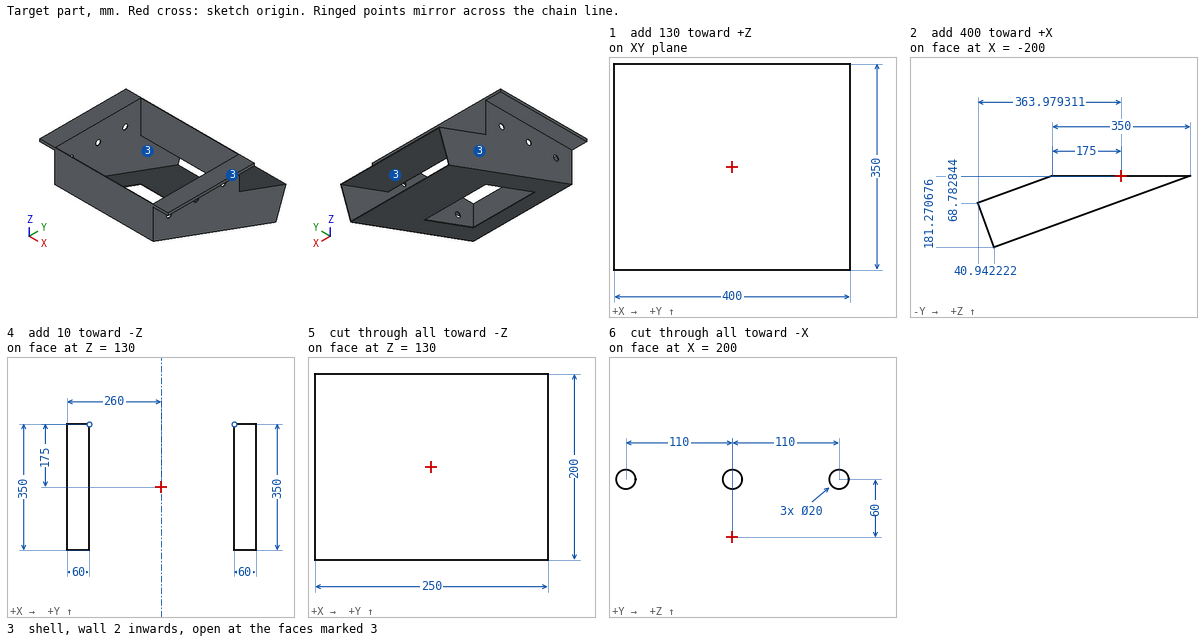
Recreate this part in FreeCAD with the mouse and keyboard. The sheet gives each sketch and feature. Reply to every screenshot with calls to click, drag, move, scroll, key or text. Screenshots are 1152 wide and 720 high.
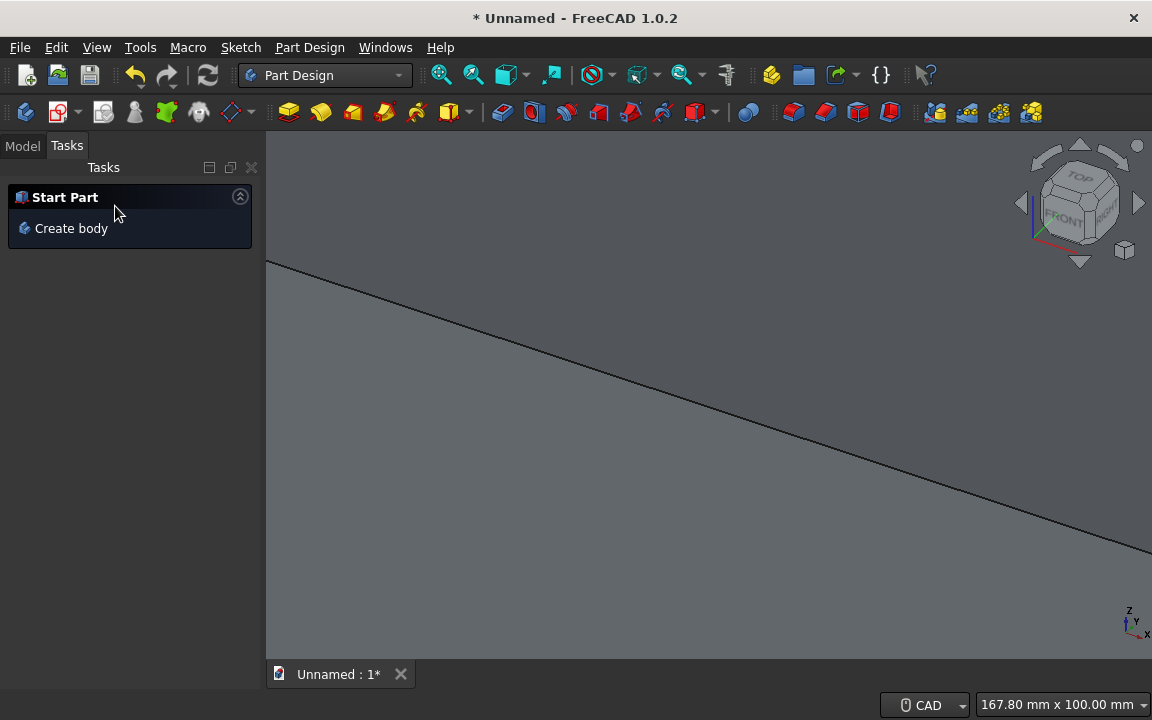
key(v)
key(f)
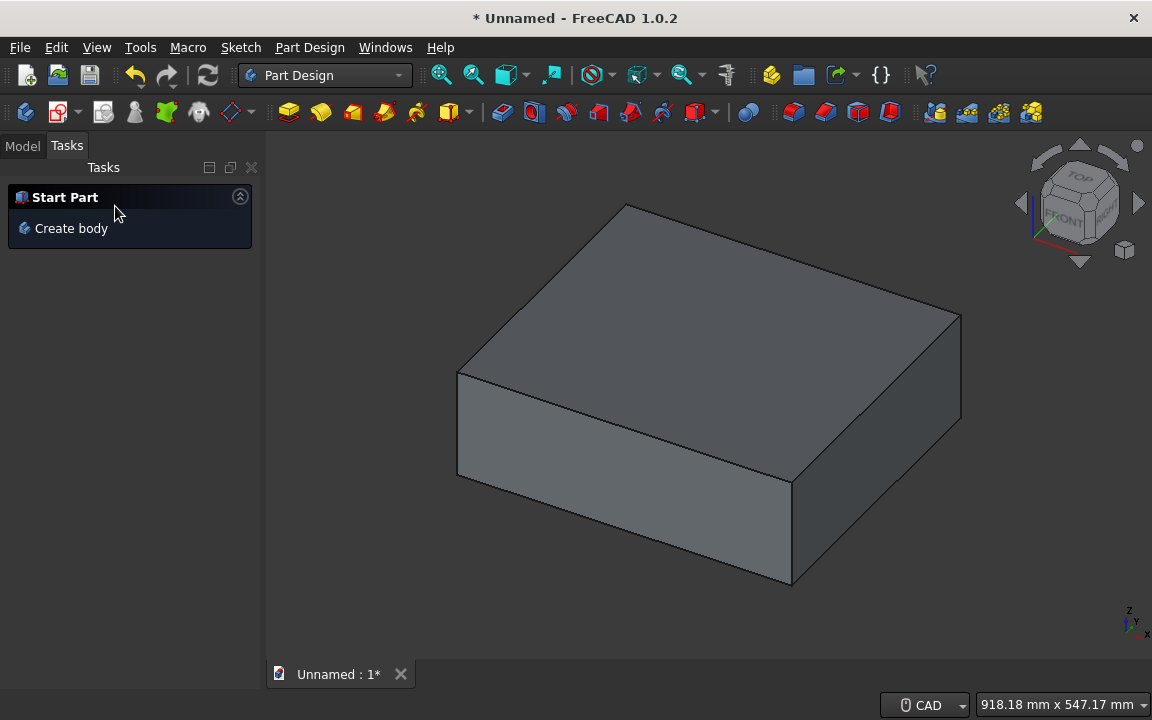
key(6)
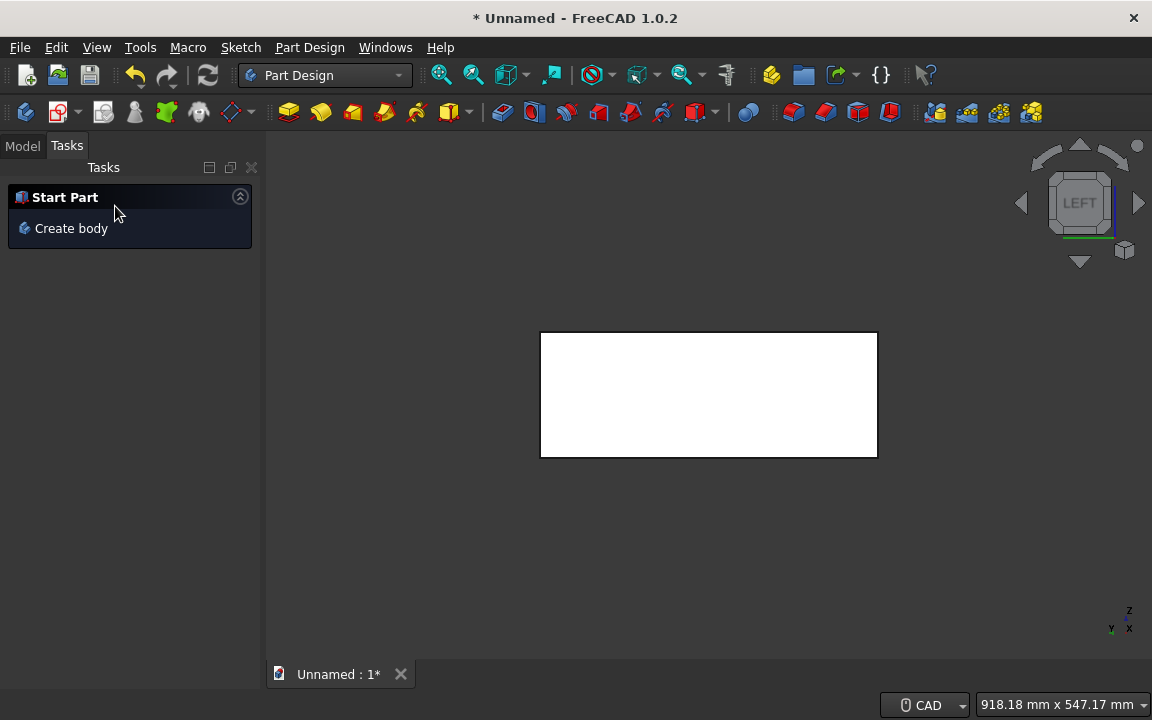
click(442, 76)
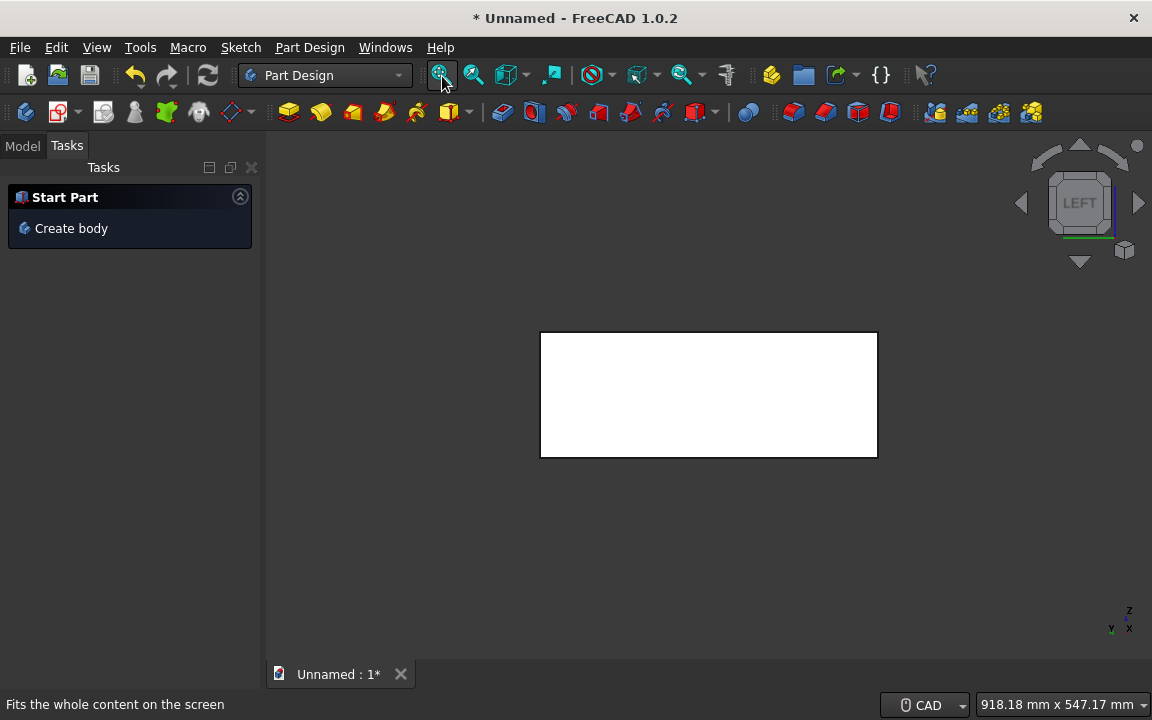
click(613, 394)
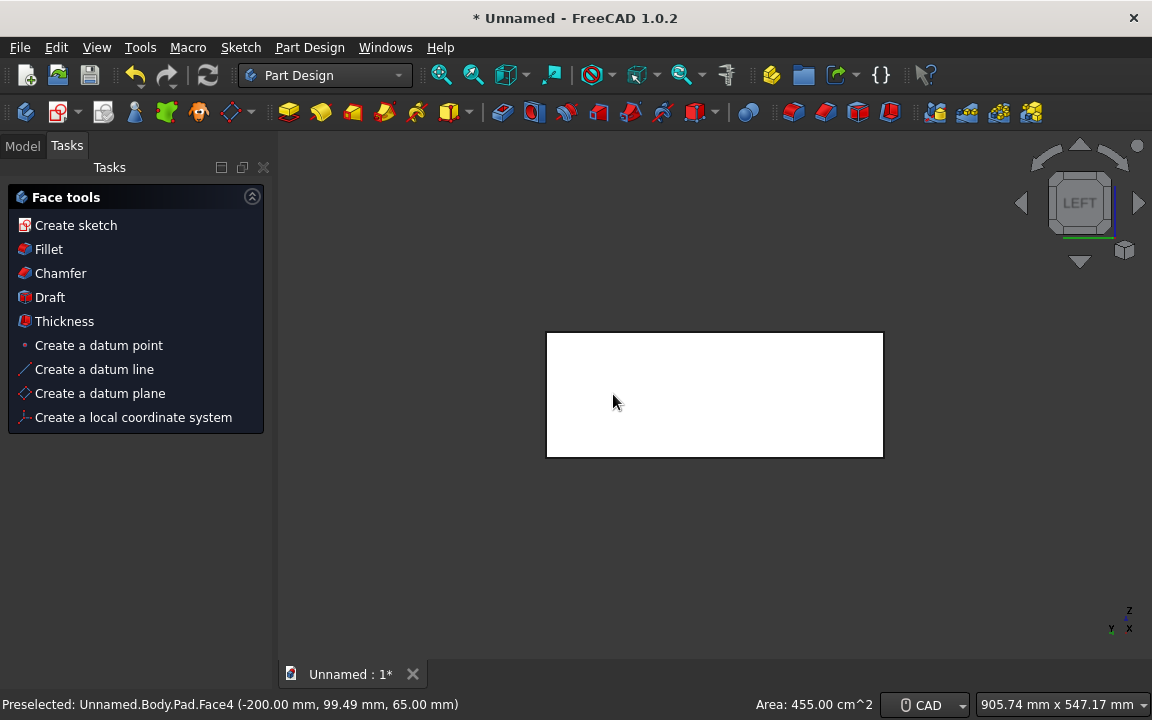
click(58, 112)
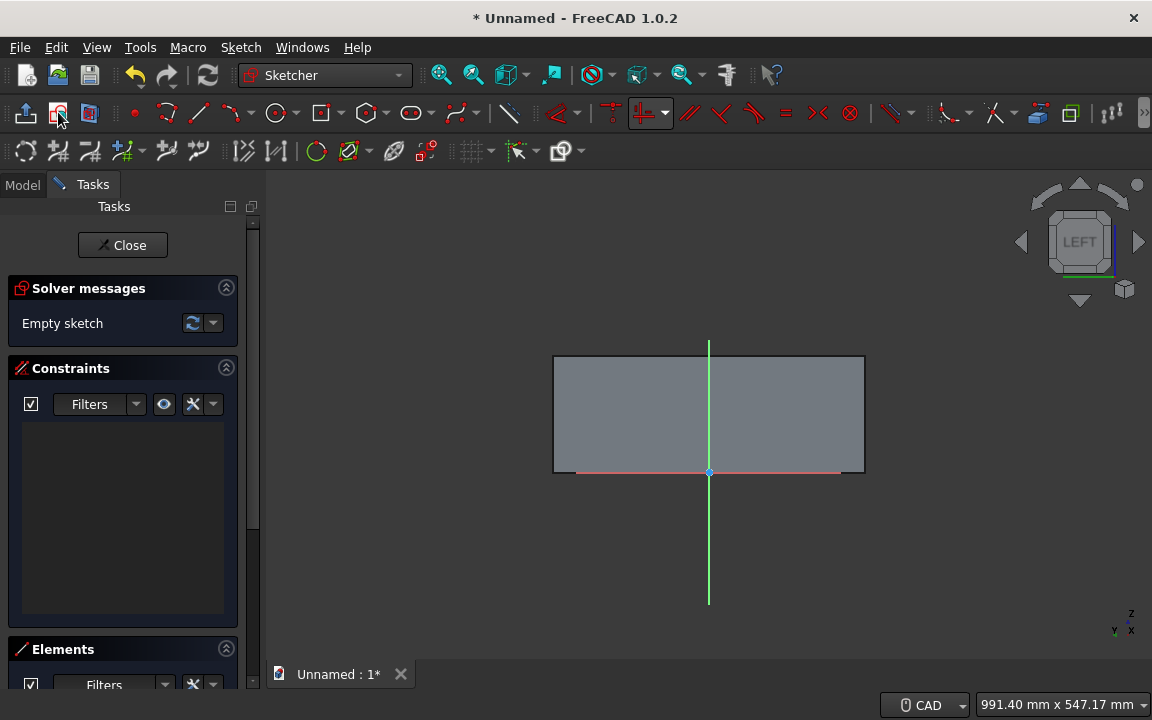
scroll(713, 198, down, 1)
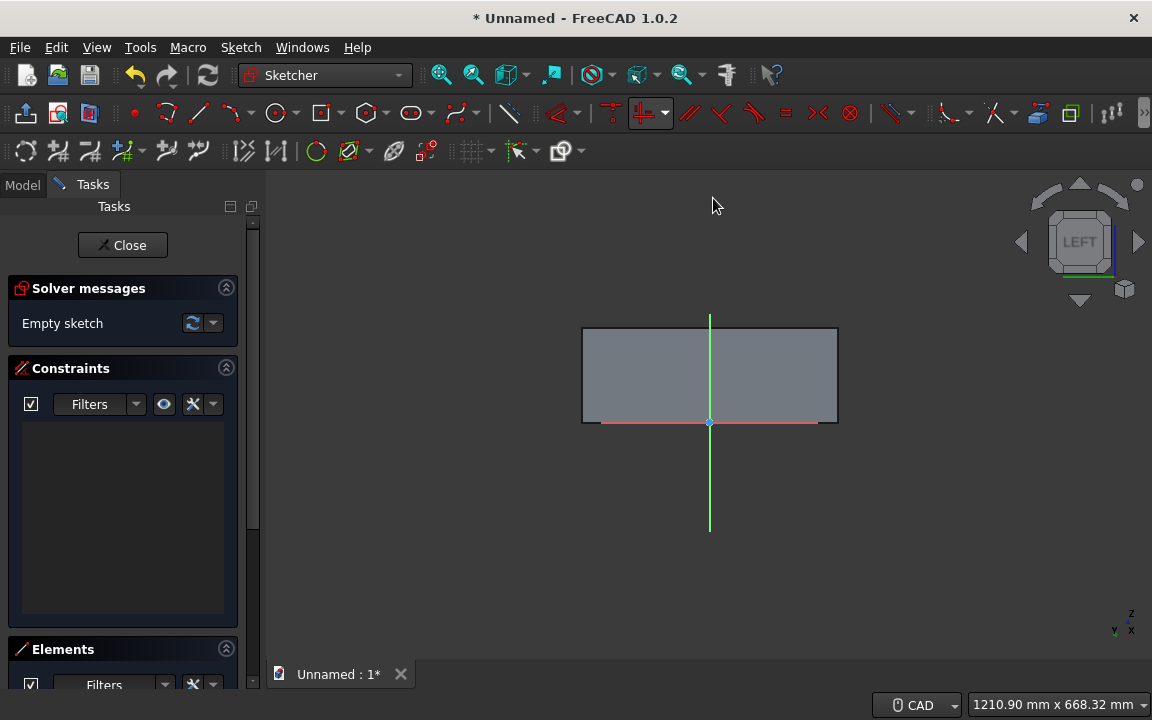
click(168, 114)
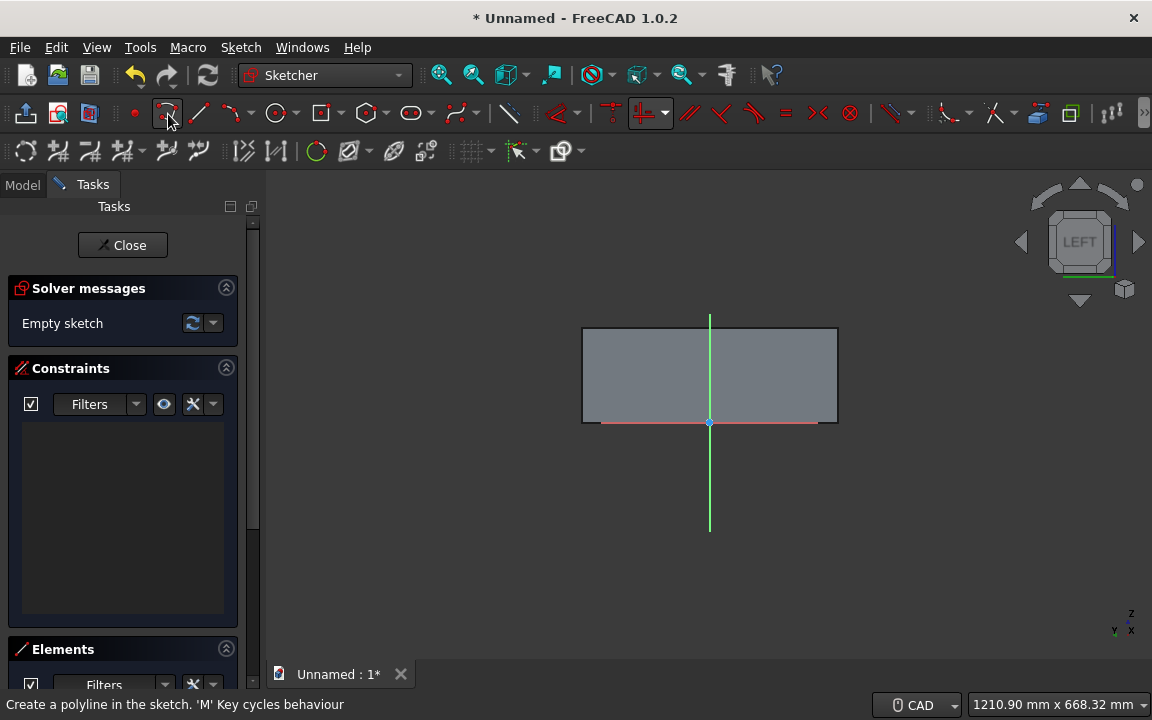
click(582, 423)
click(443, 473)
click(473, 555)
click(838, 432)
click(582, 424)
key(Escape)
key(Escape)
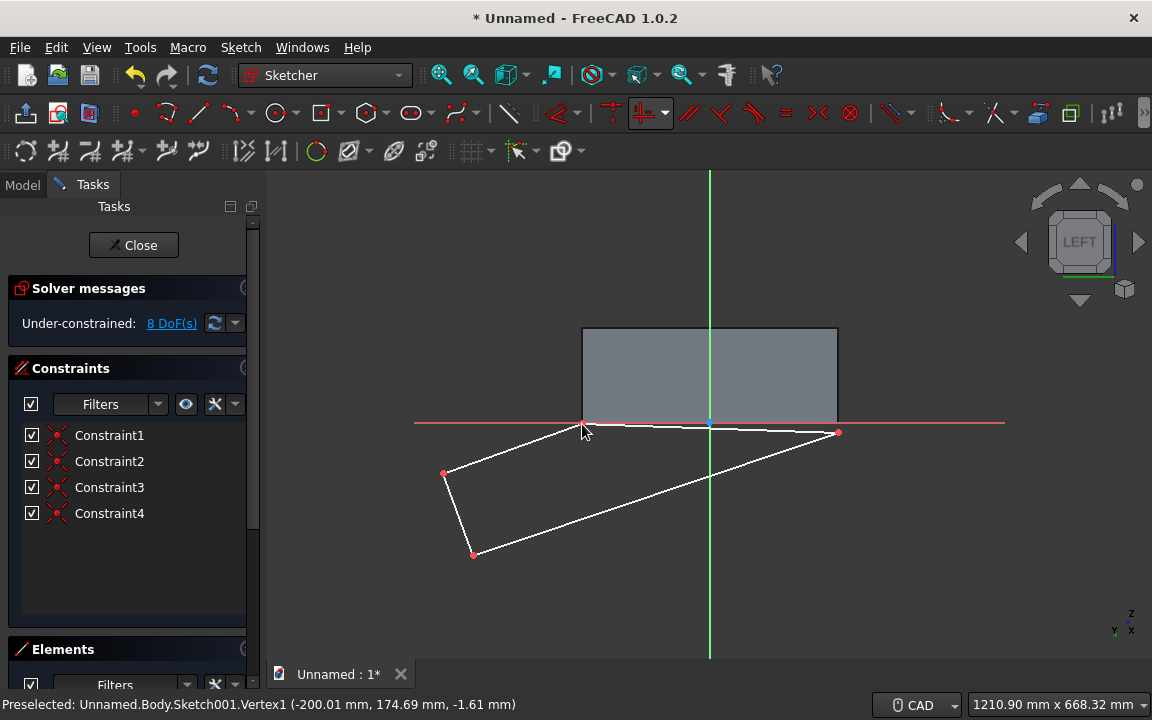
click(659, 427)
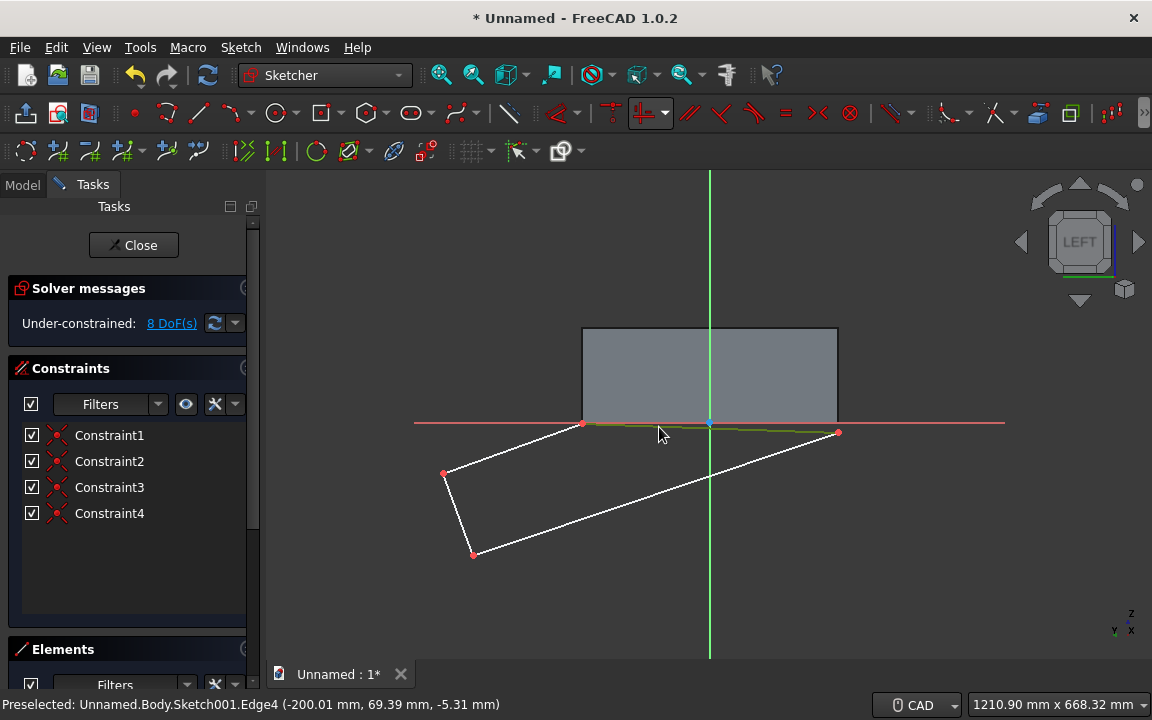
key(h)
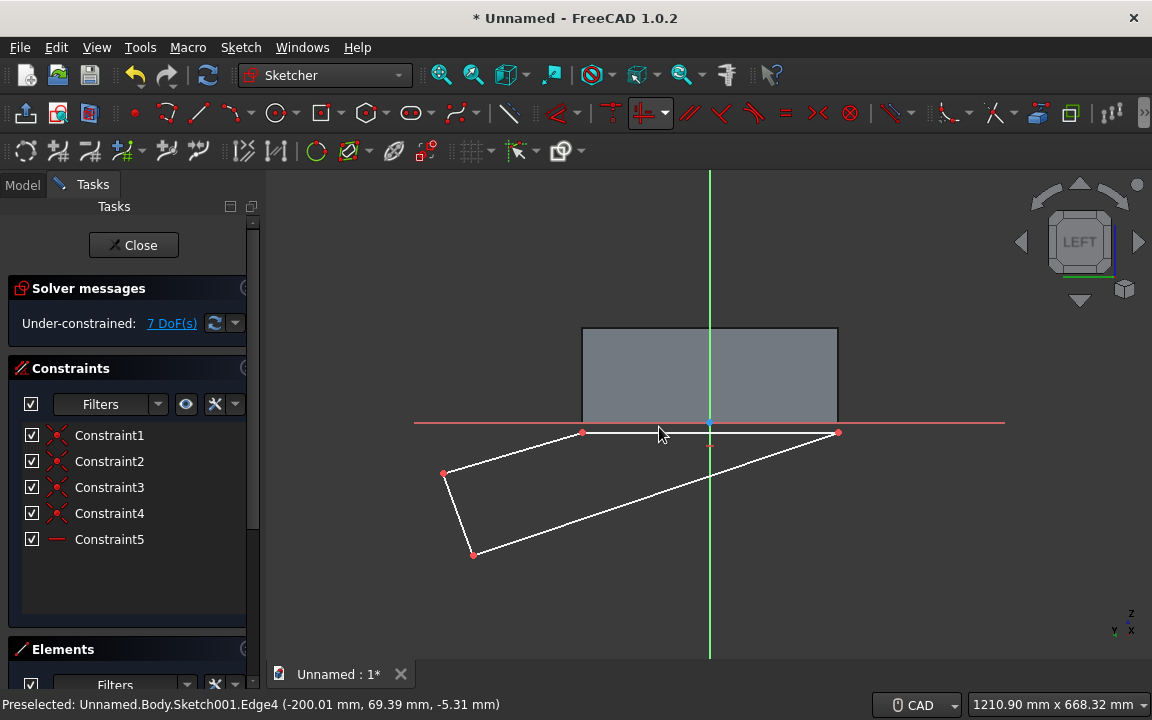
click(582, 433)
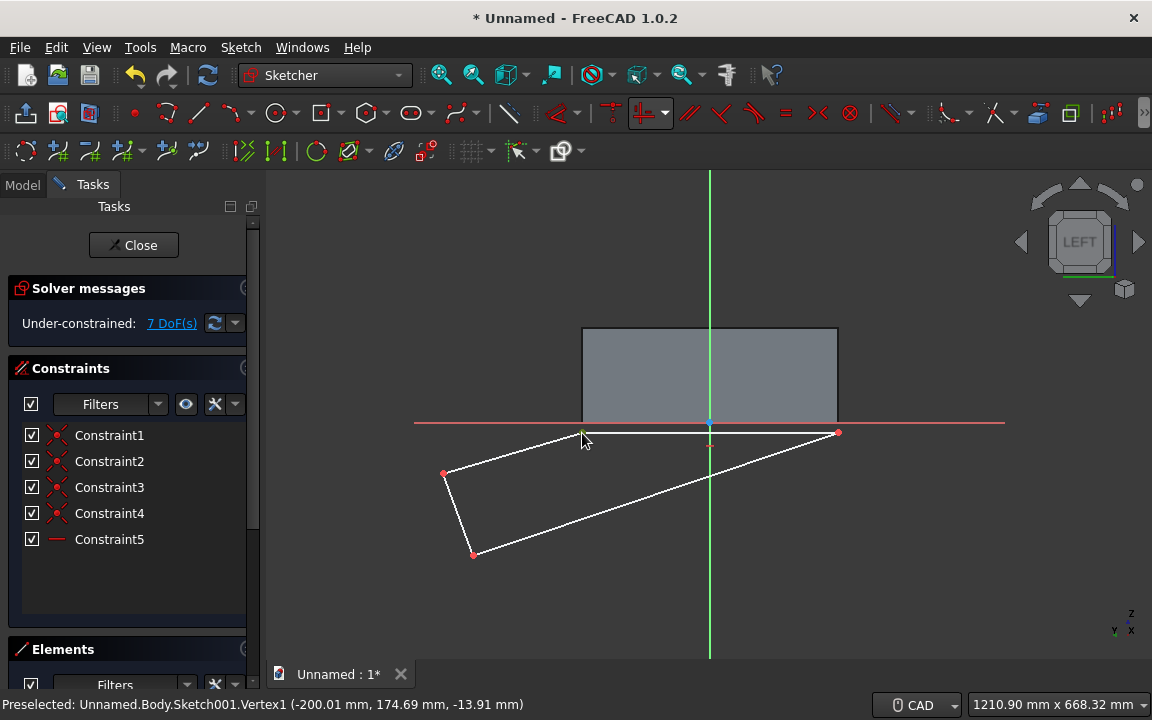
click(442, 423)